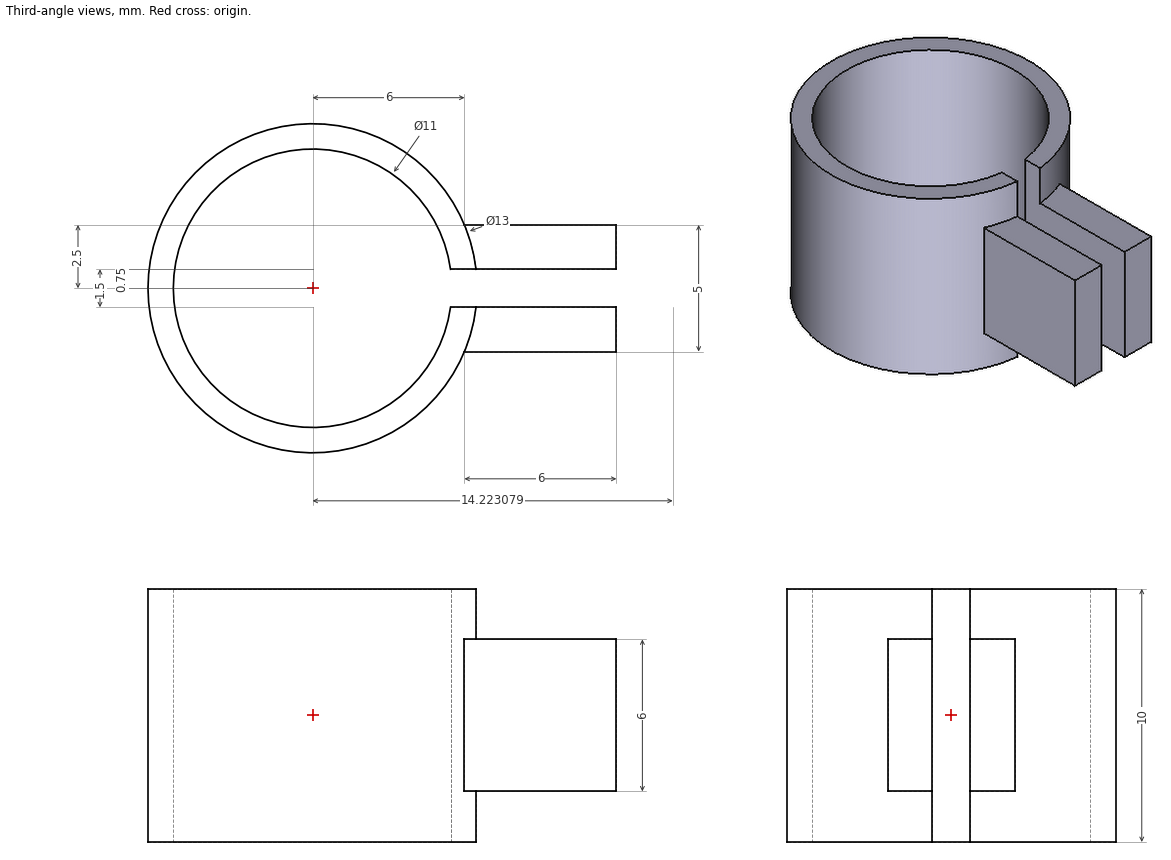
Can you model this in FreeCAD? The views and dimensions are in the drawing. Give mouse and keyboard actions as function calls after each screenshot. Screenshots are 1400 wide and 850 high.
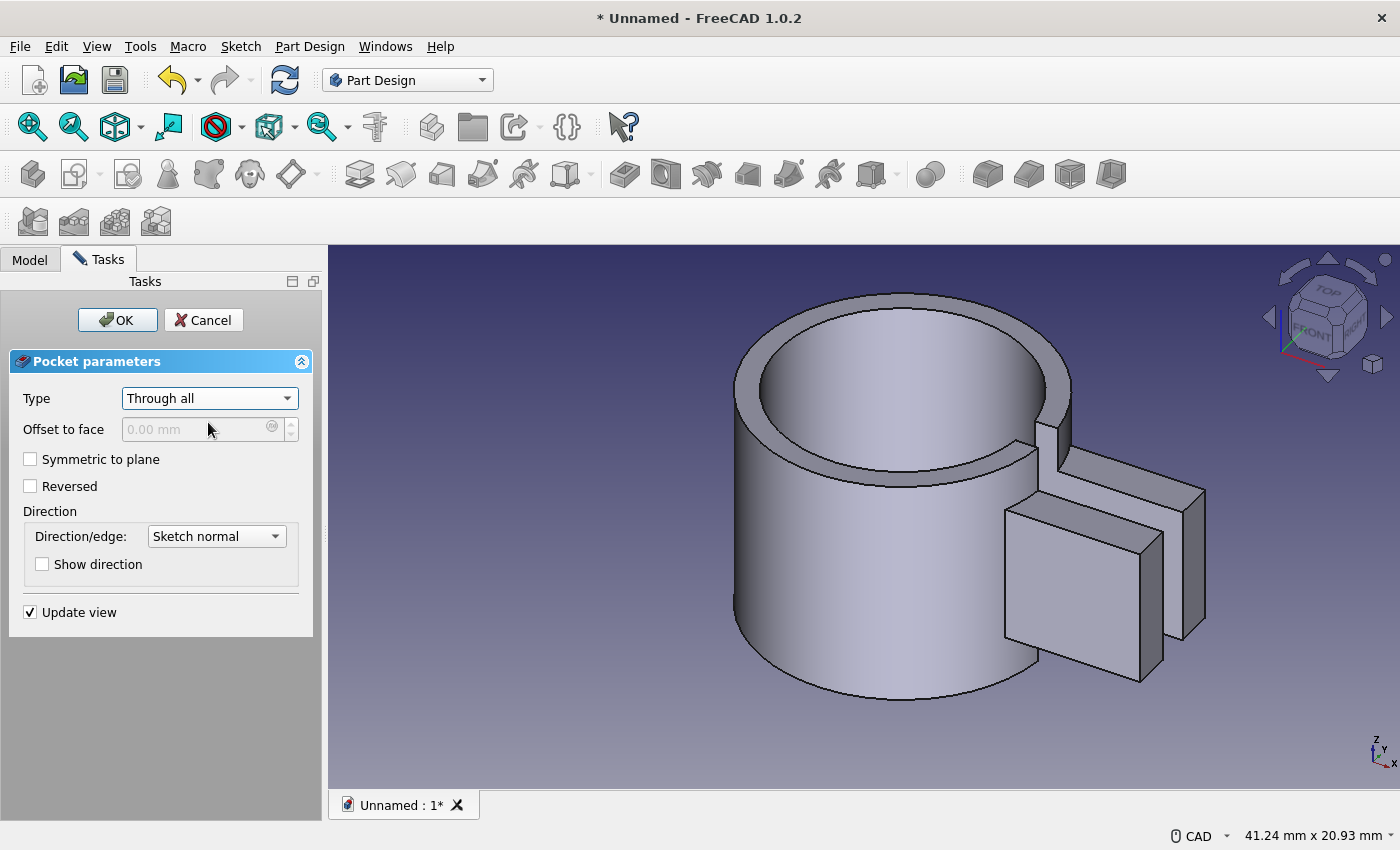
click(118, 320)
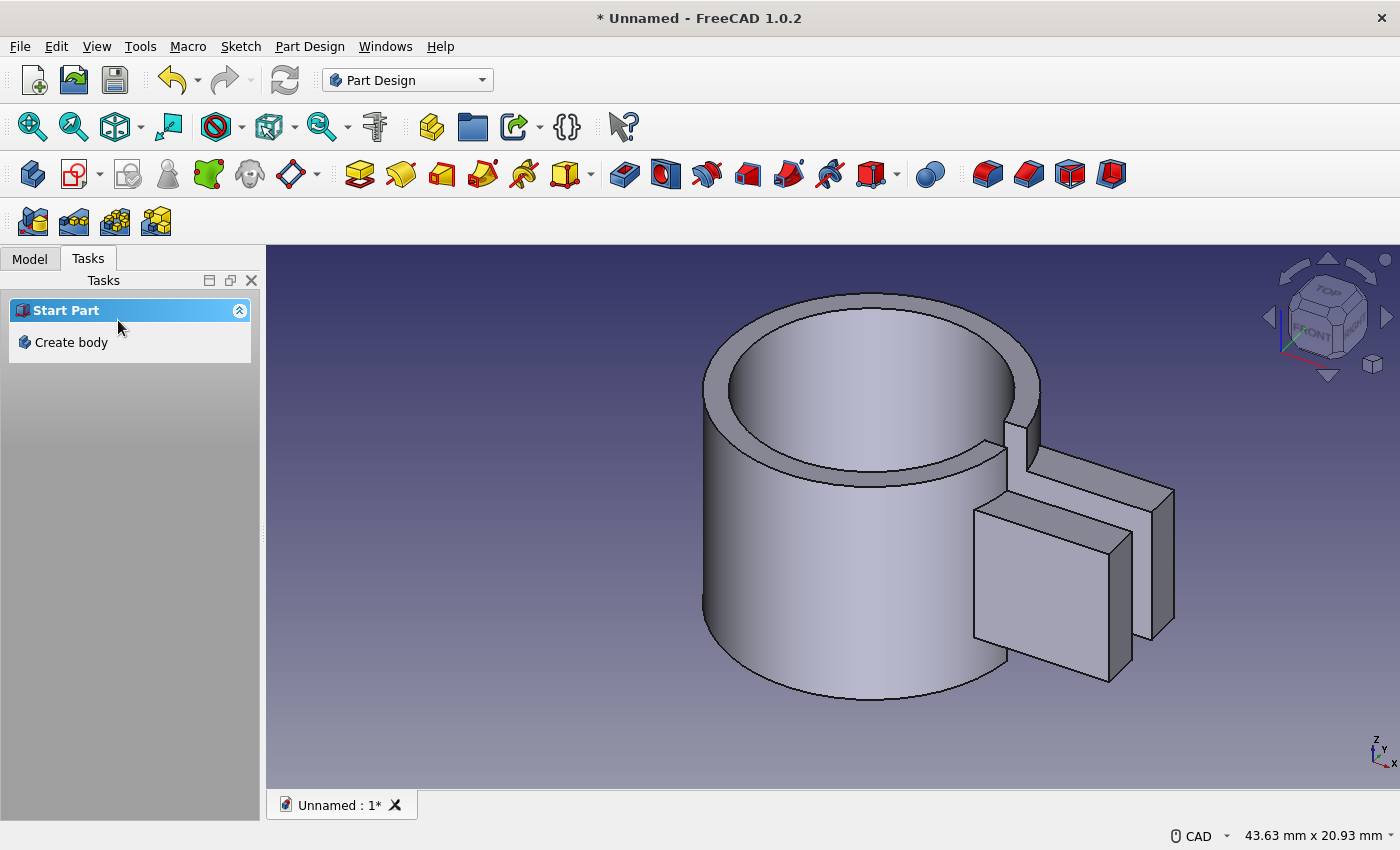
key(0)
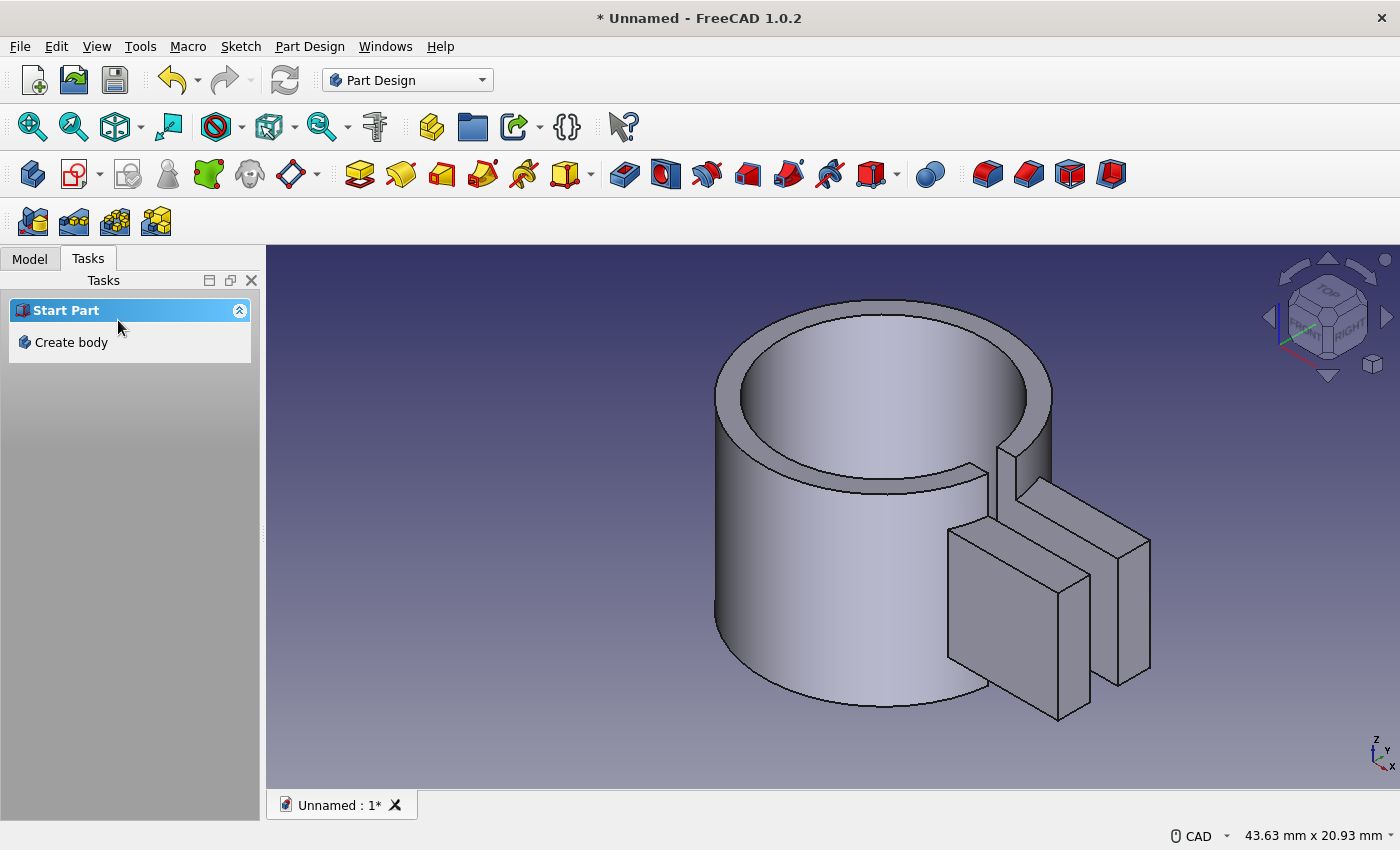
key(v)
key(f)